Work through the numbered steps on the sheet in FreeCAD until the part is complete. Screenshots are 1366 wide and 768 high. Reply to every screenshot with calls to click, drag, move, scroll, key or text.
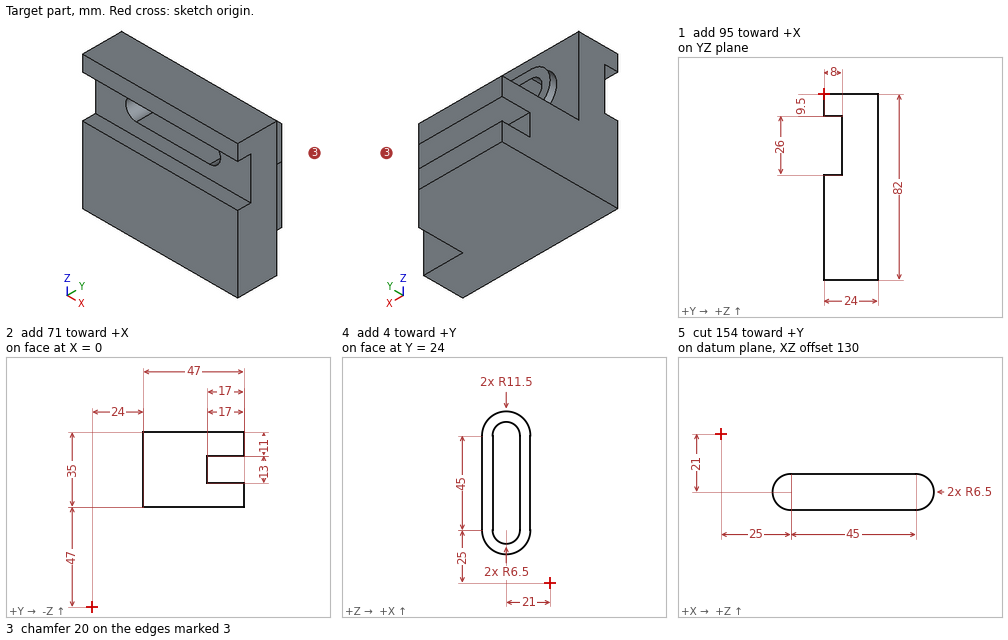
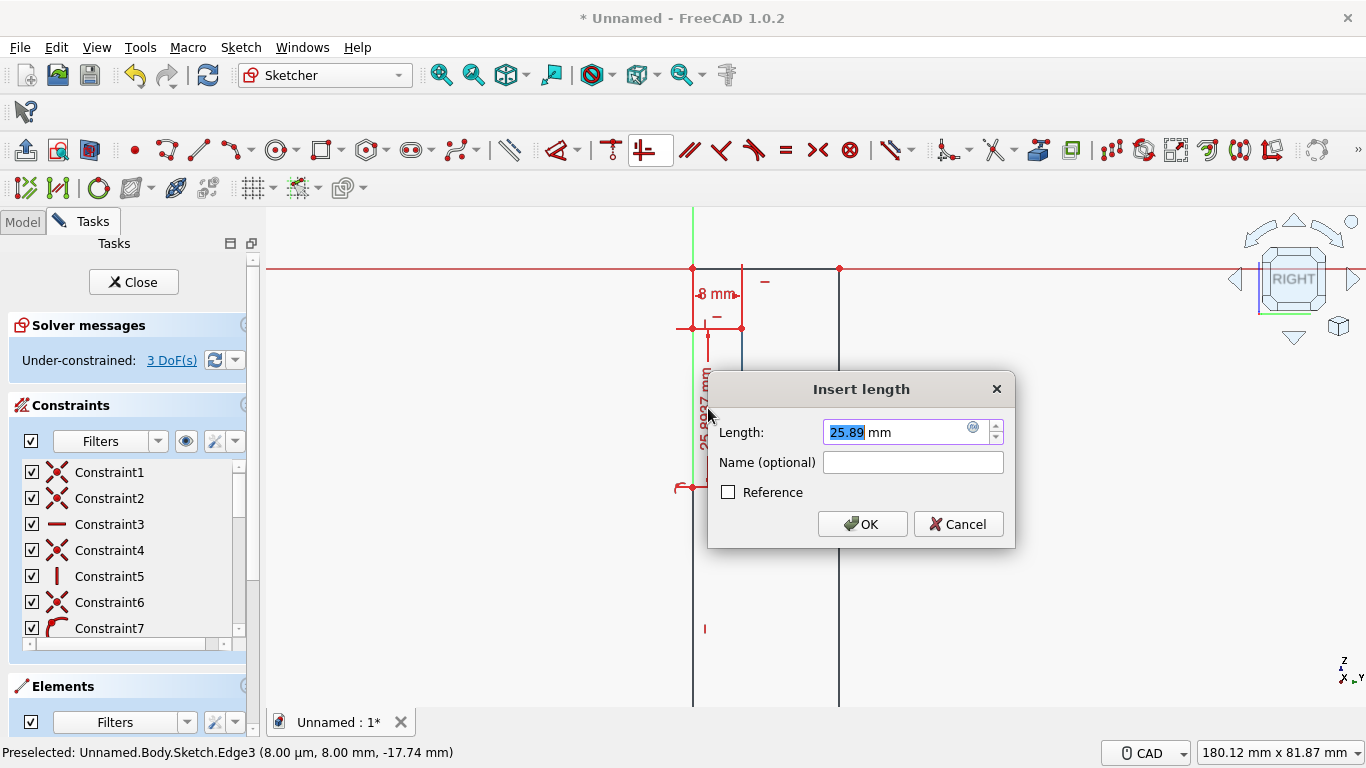
text(26)
key(Return)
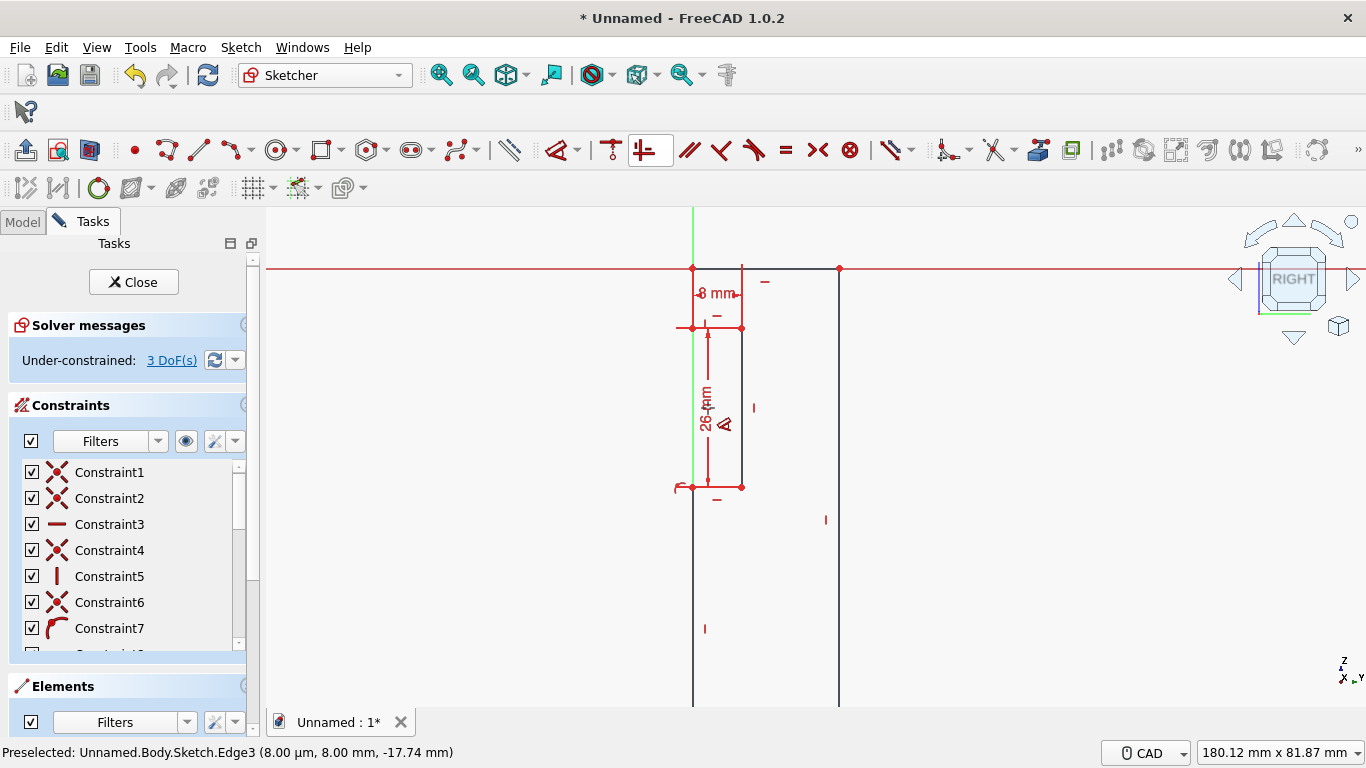
scroll(710, 331, down, 2)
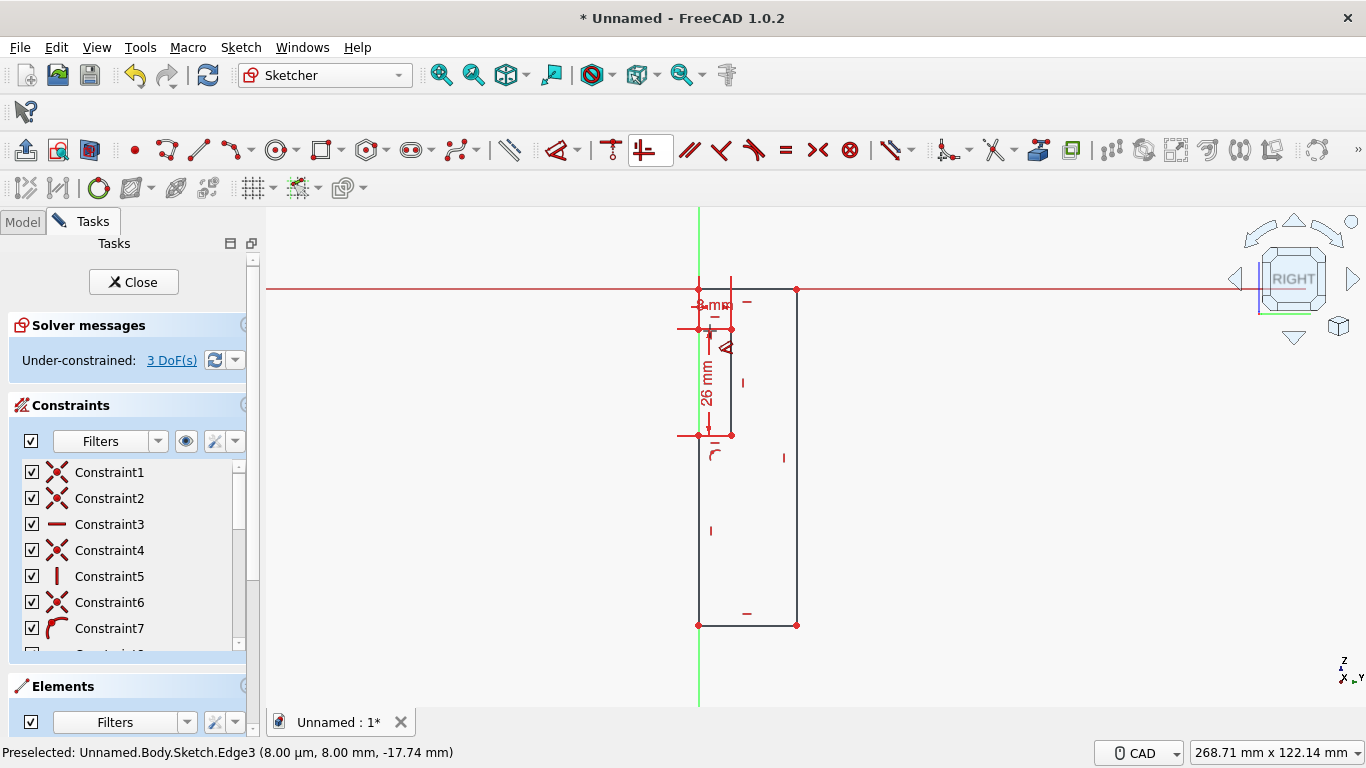
click(728, 626)
click(748, 660)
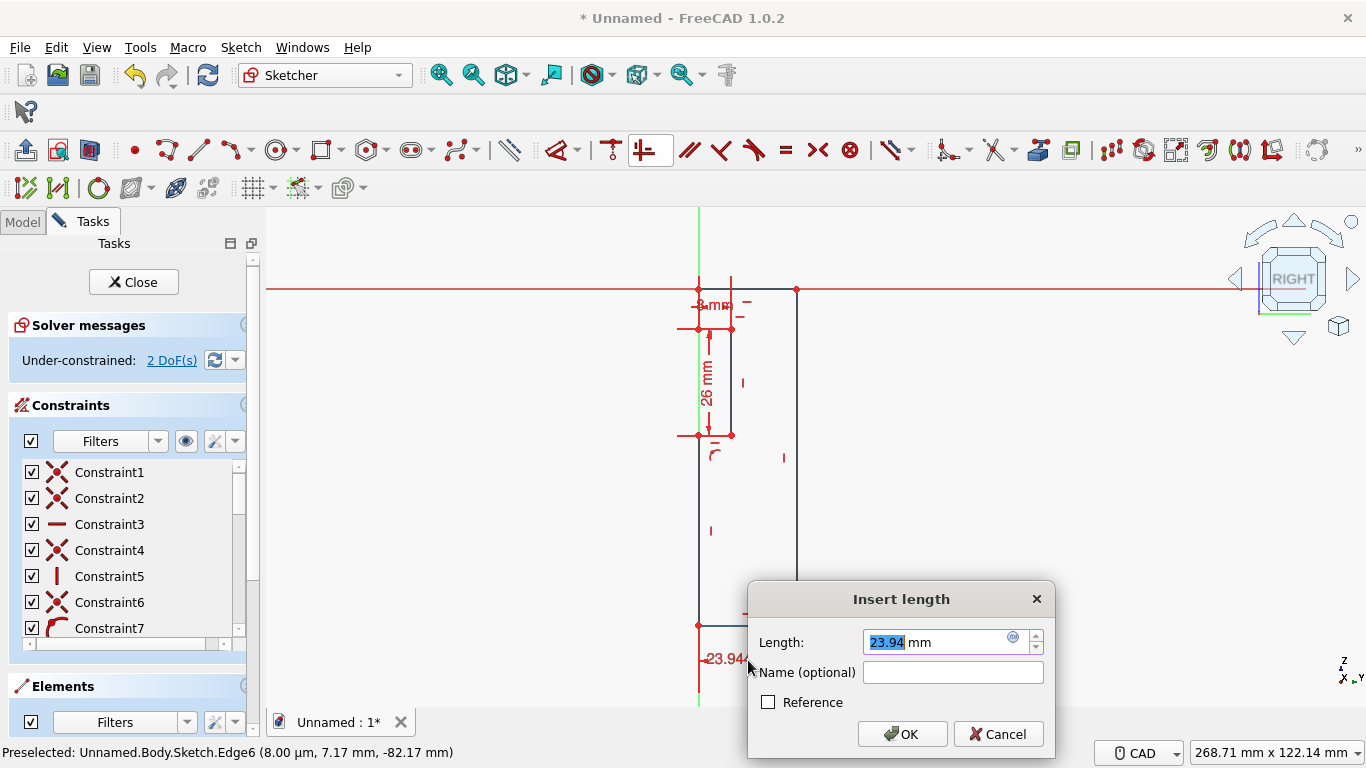
text(24)
key(Return)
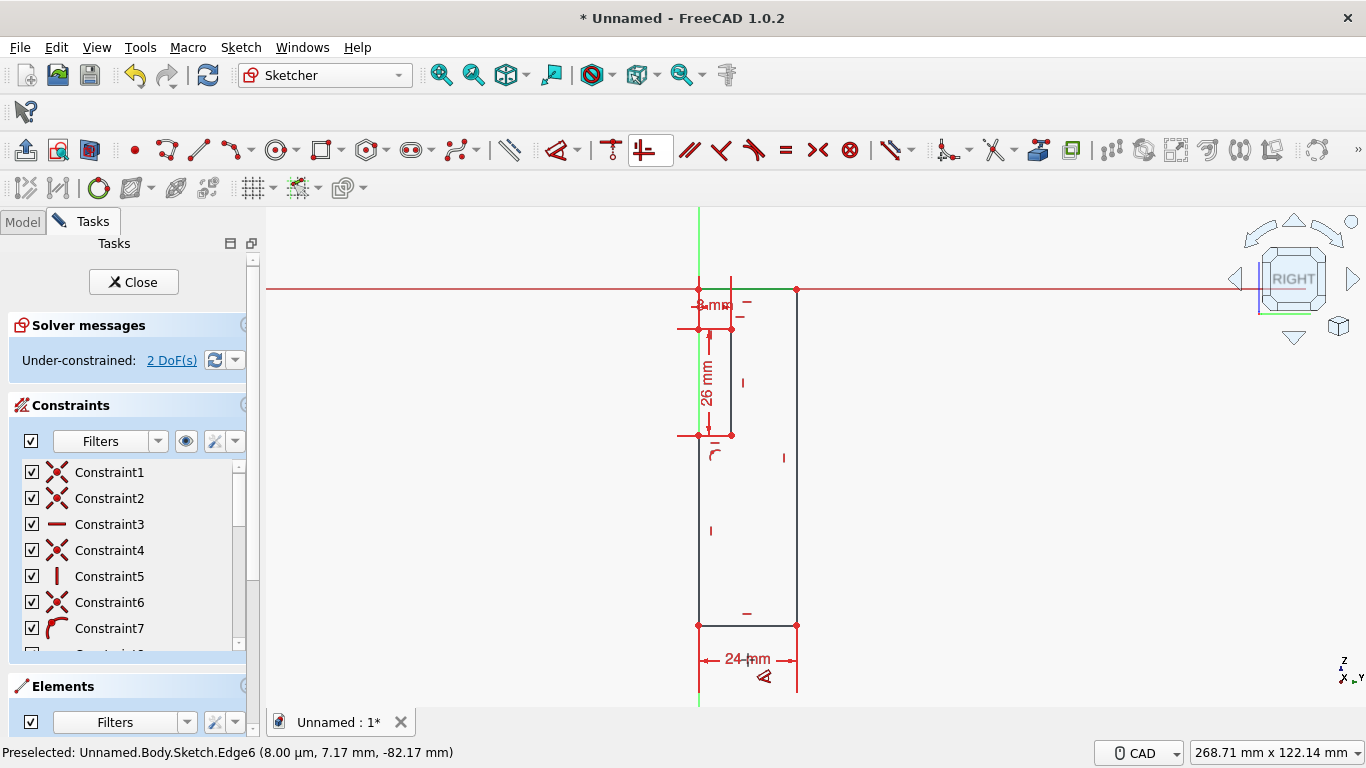
click(797, 525)
click(831, 457)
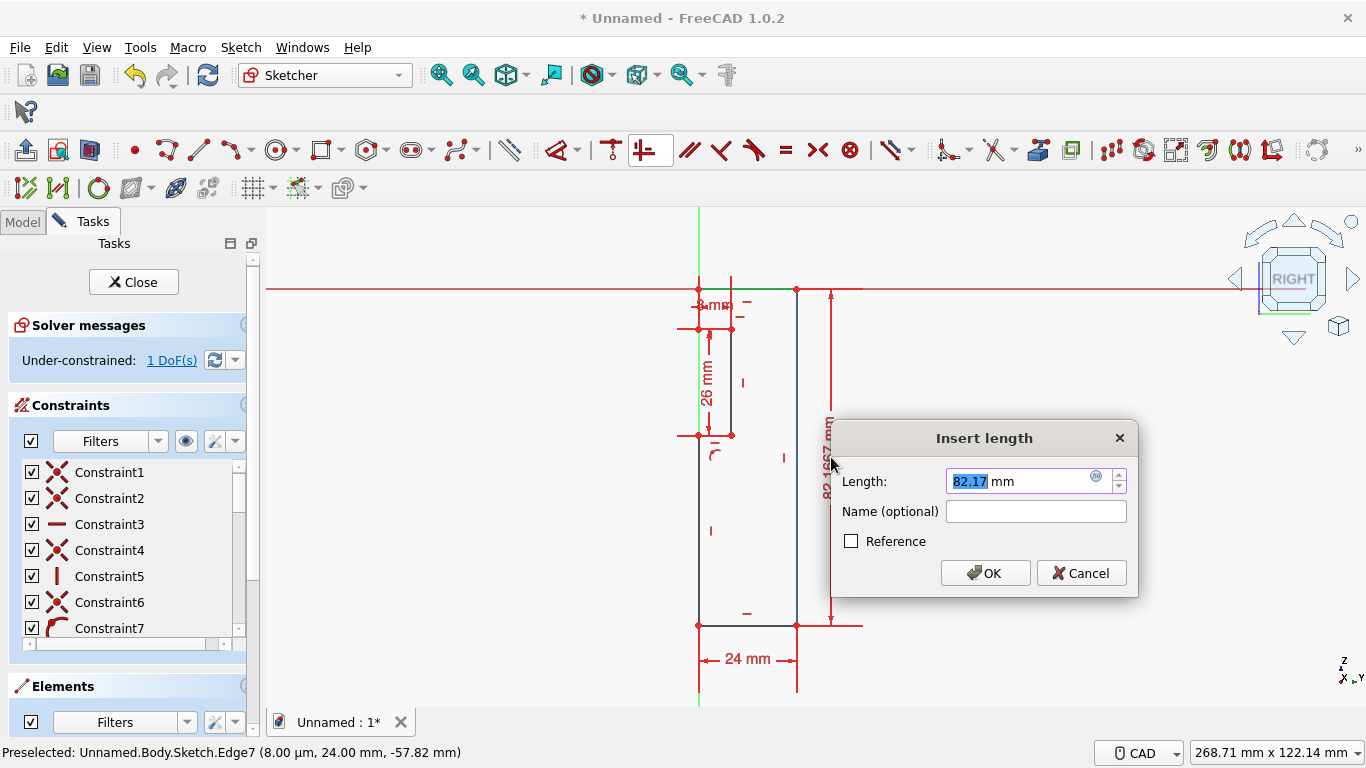
text(82)
key(Return)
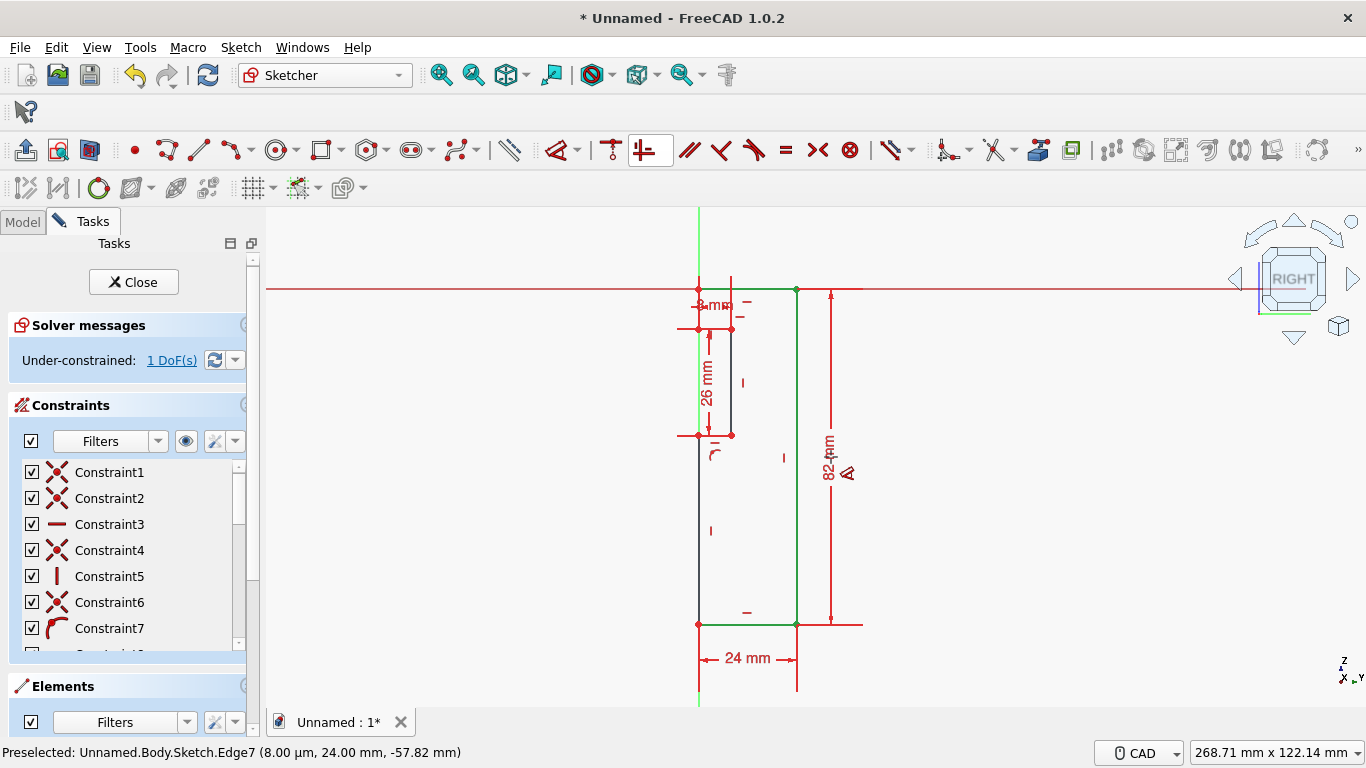
click(699, 301)
click(641, 309)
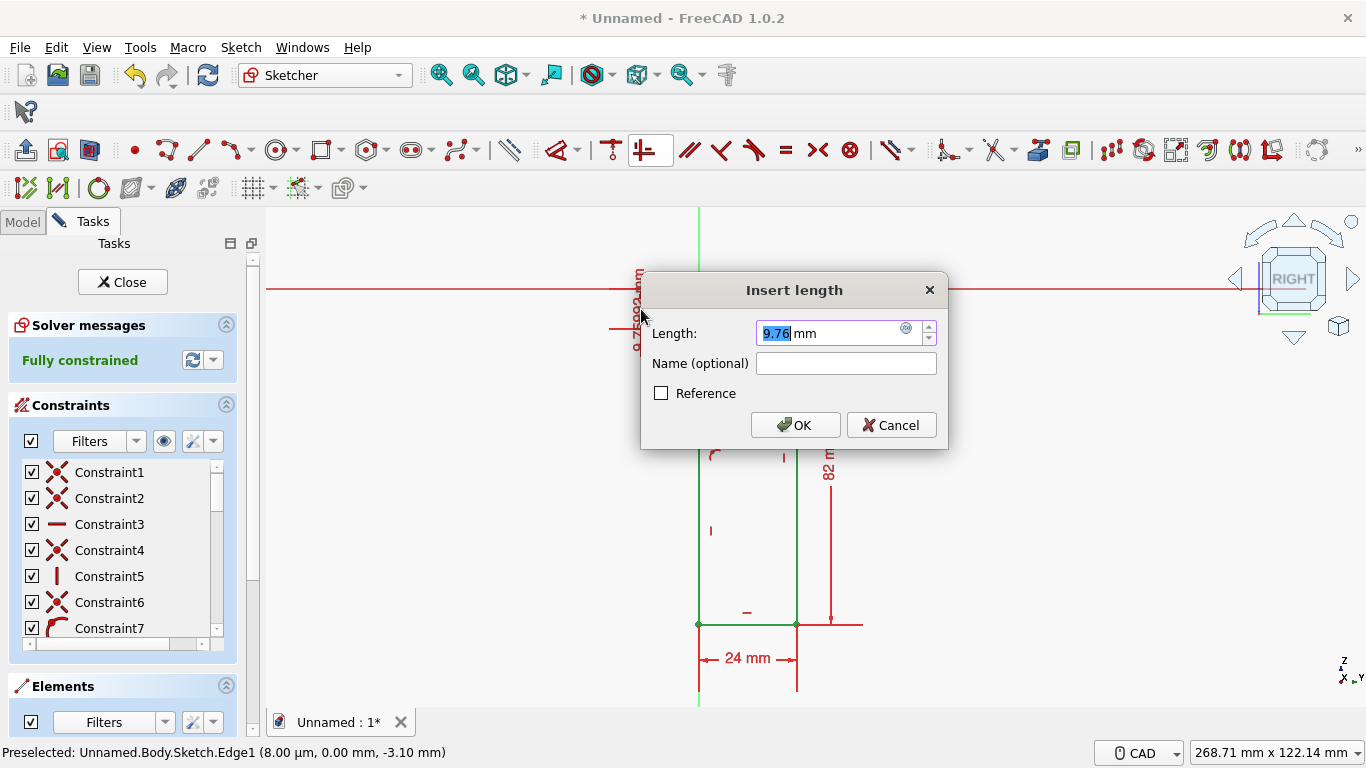
text(9.5)
key(Return)
key(Escape)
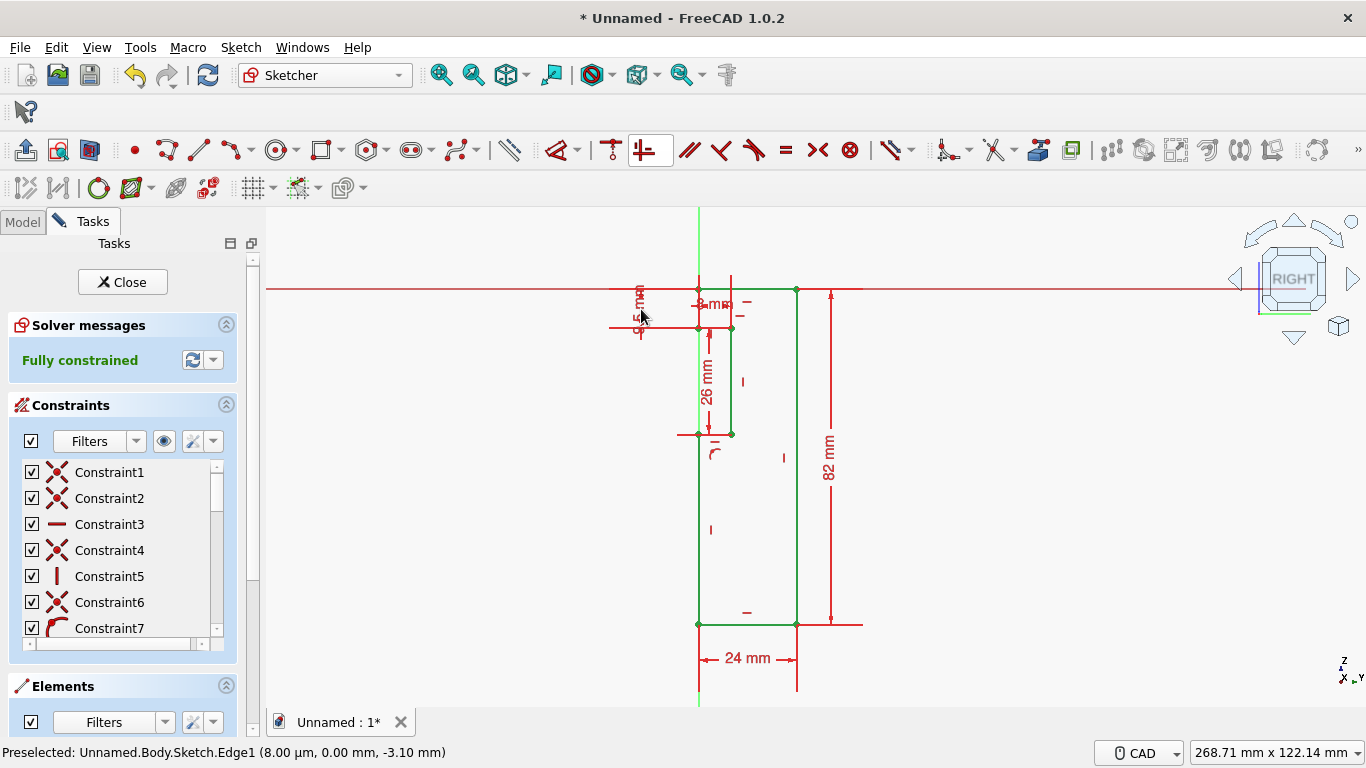
click(123, 282)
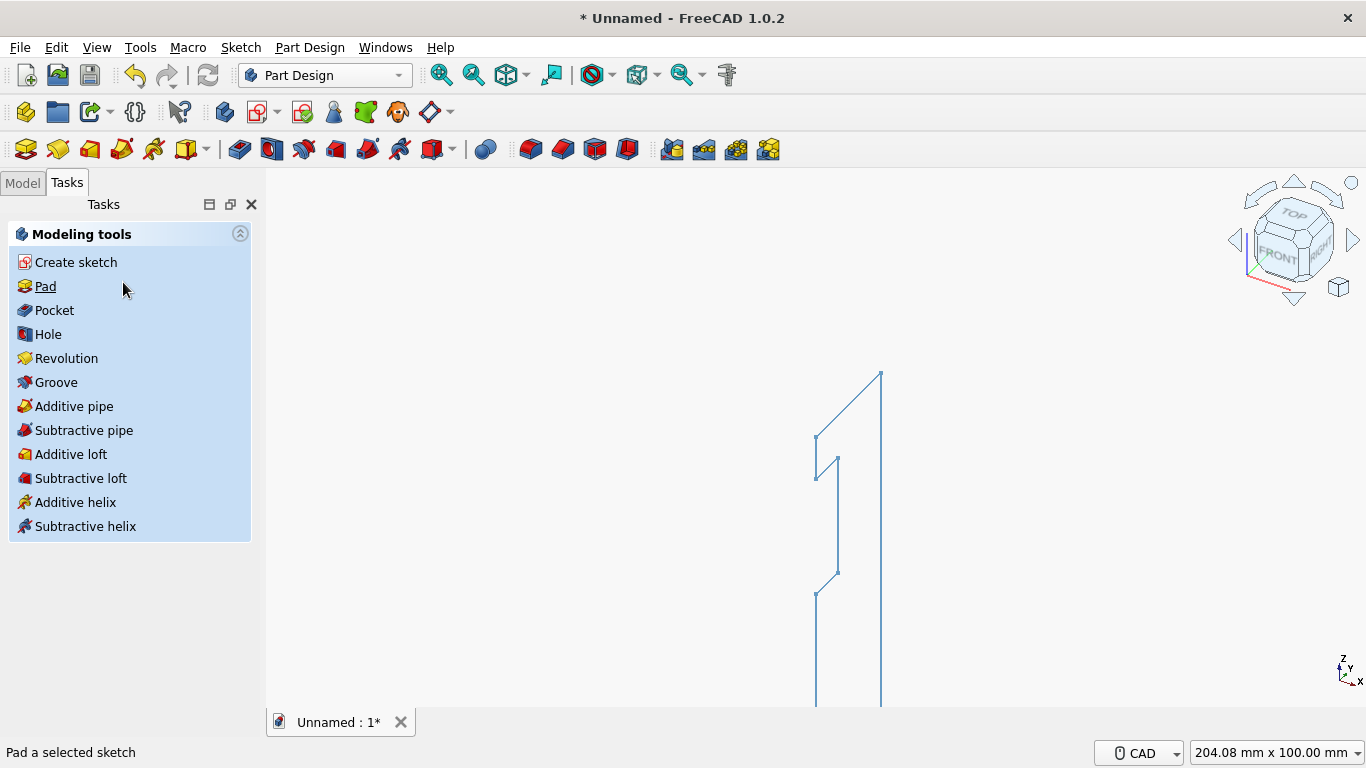
click(26, 150)